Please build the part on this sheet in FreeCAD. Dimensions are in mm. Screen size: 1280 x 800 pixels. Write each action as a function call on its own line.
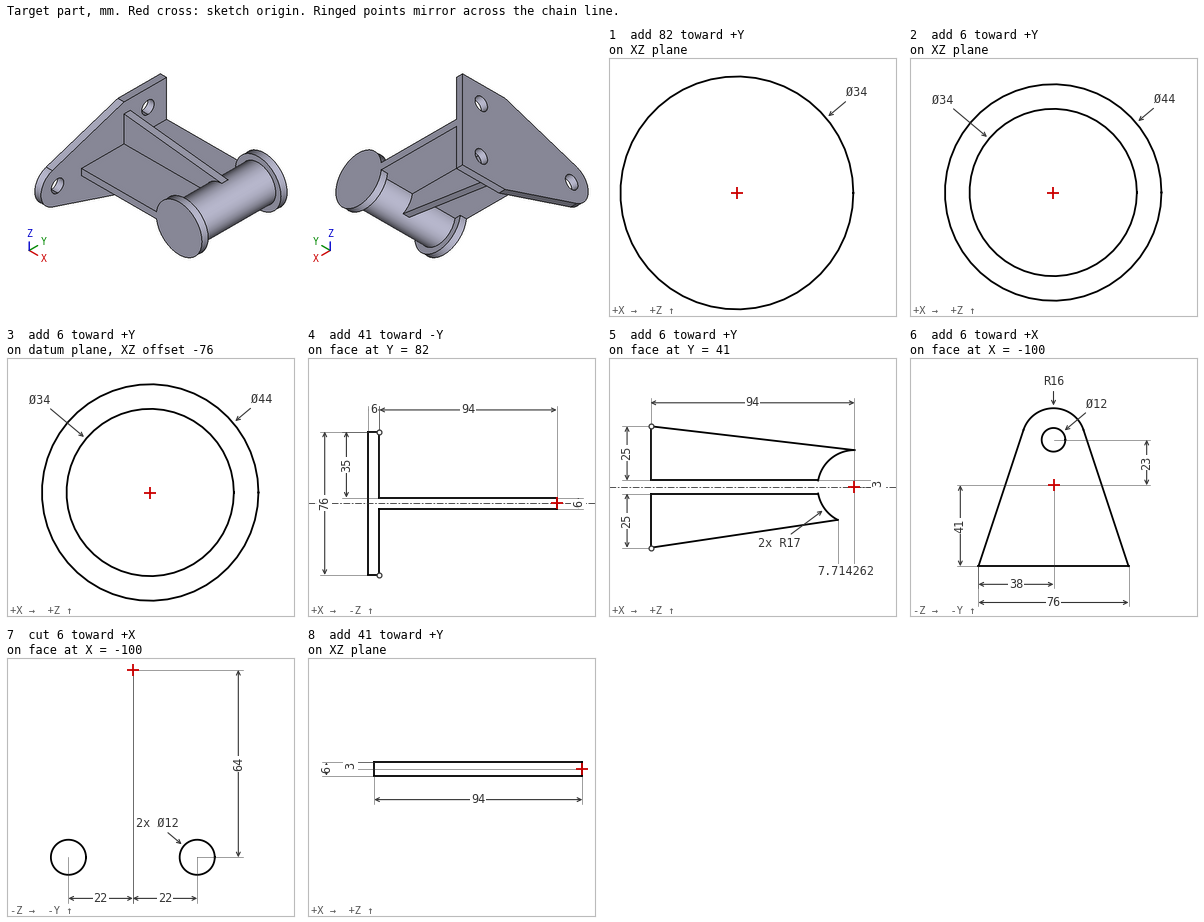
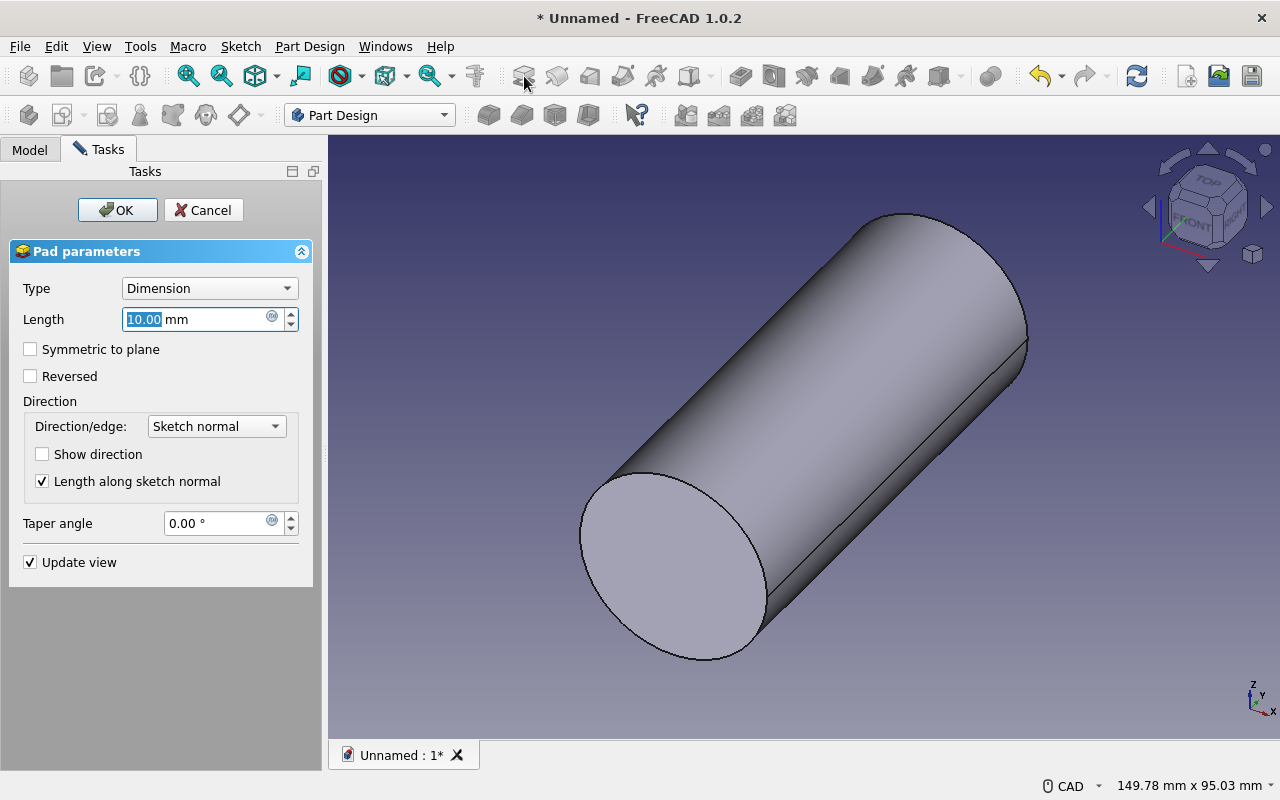
text(6)
key(Tab)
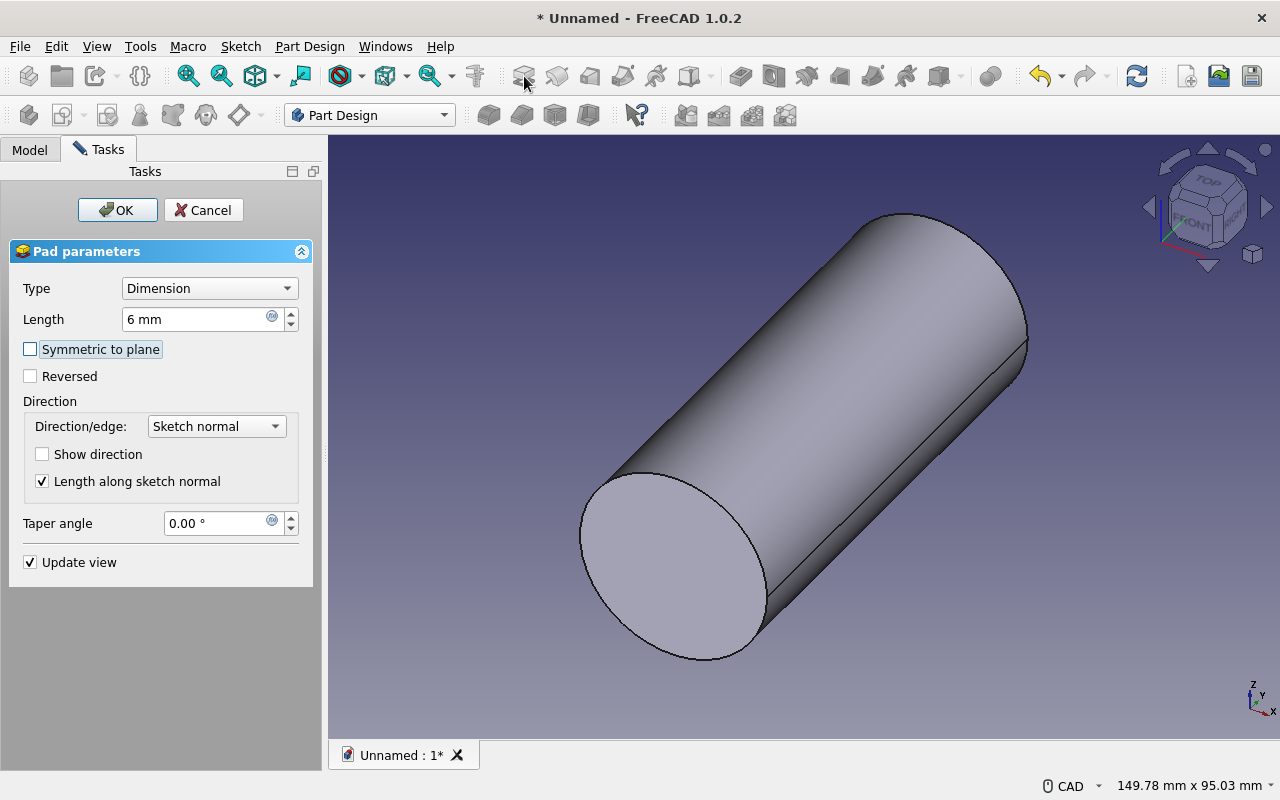
click(31, 376)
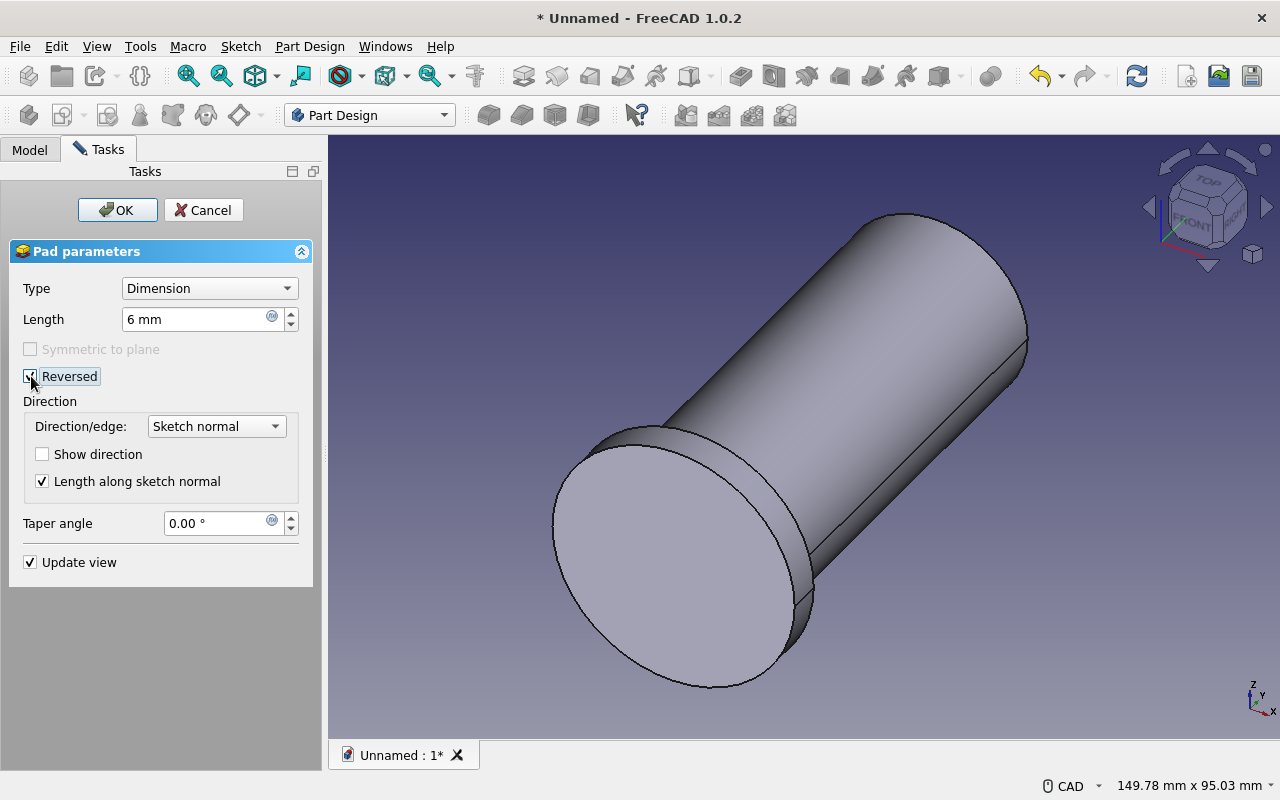
click(118, 210)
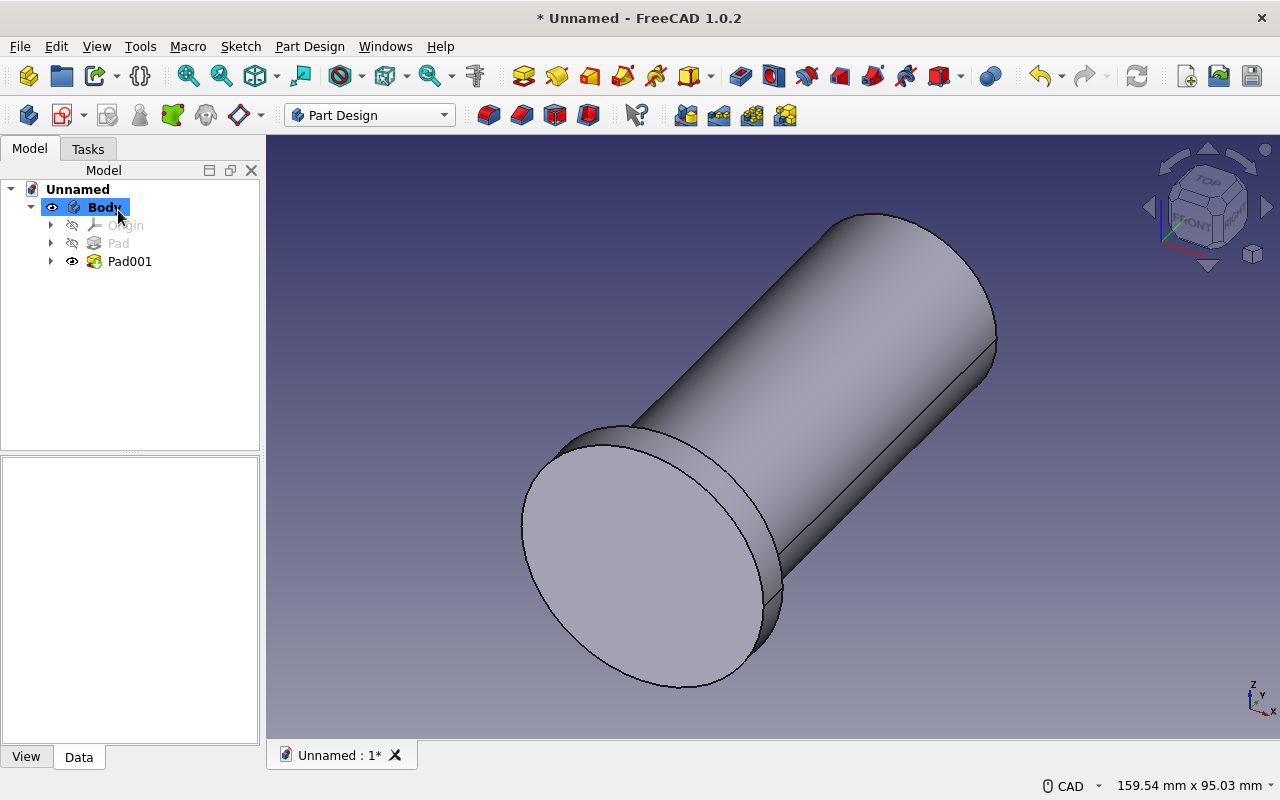
click(51, 225)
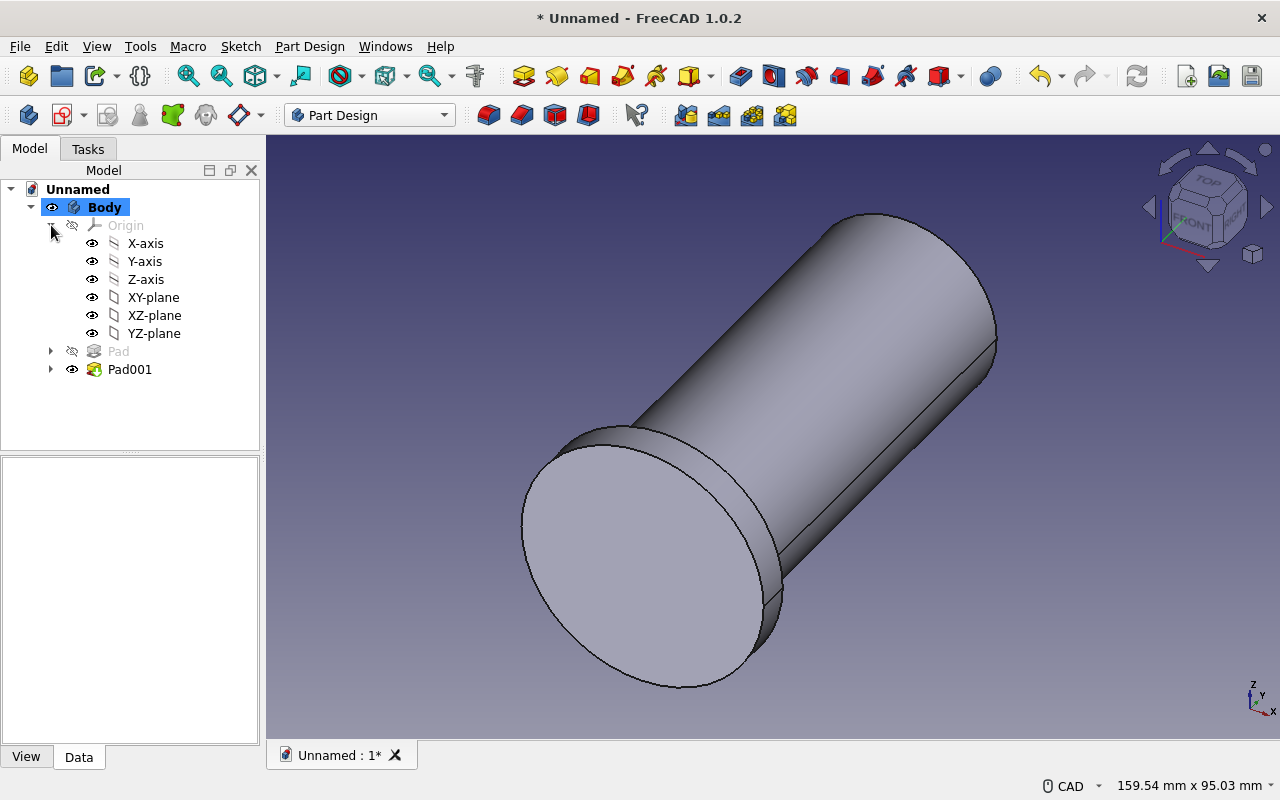
click(137, 315)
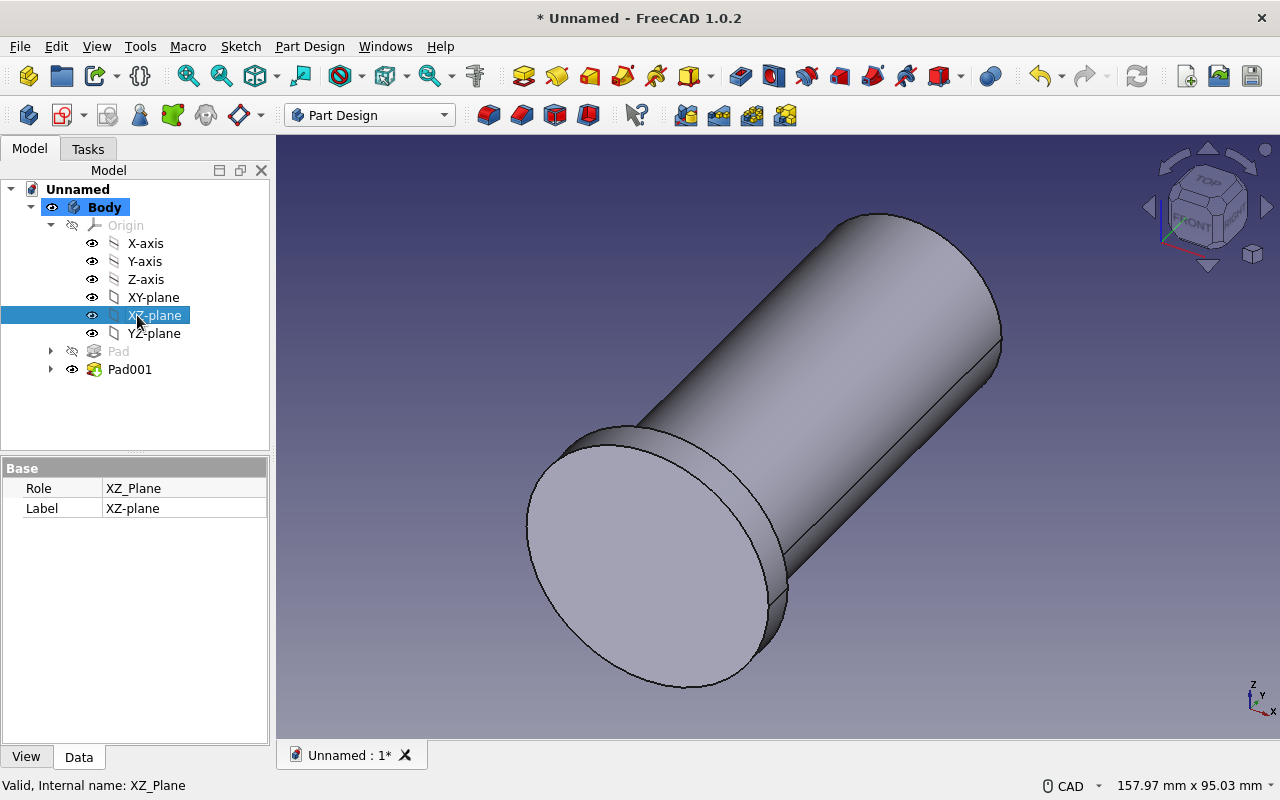
click(238, 116)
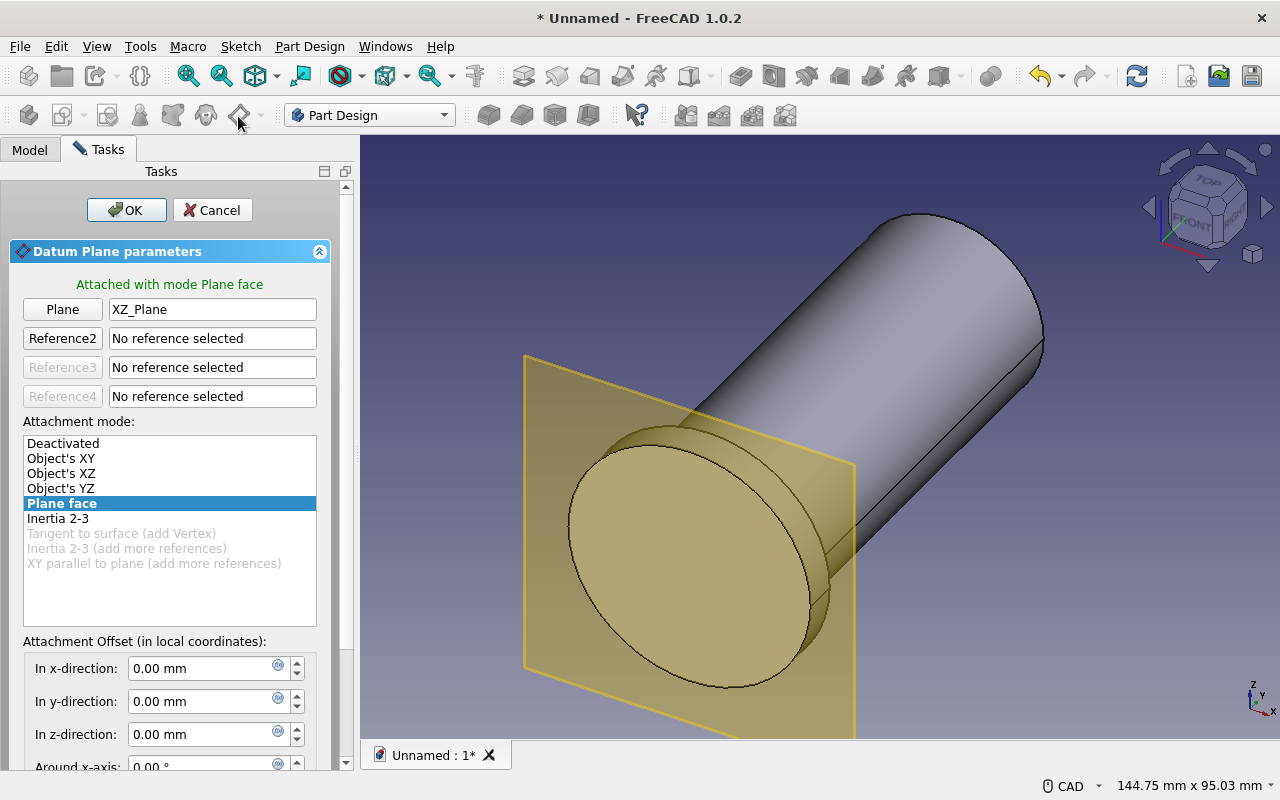
triple_click(210, 734)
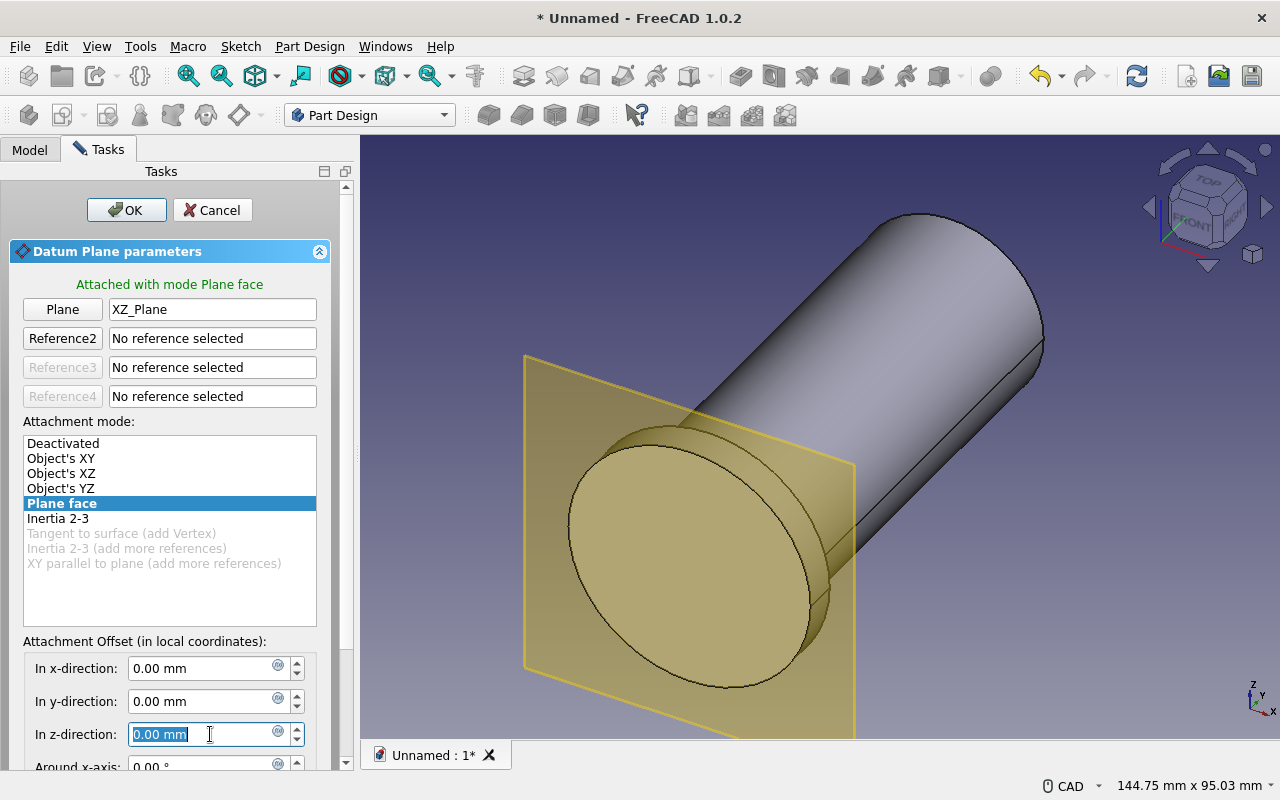
text(-76)
key(Tab)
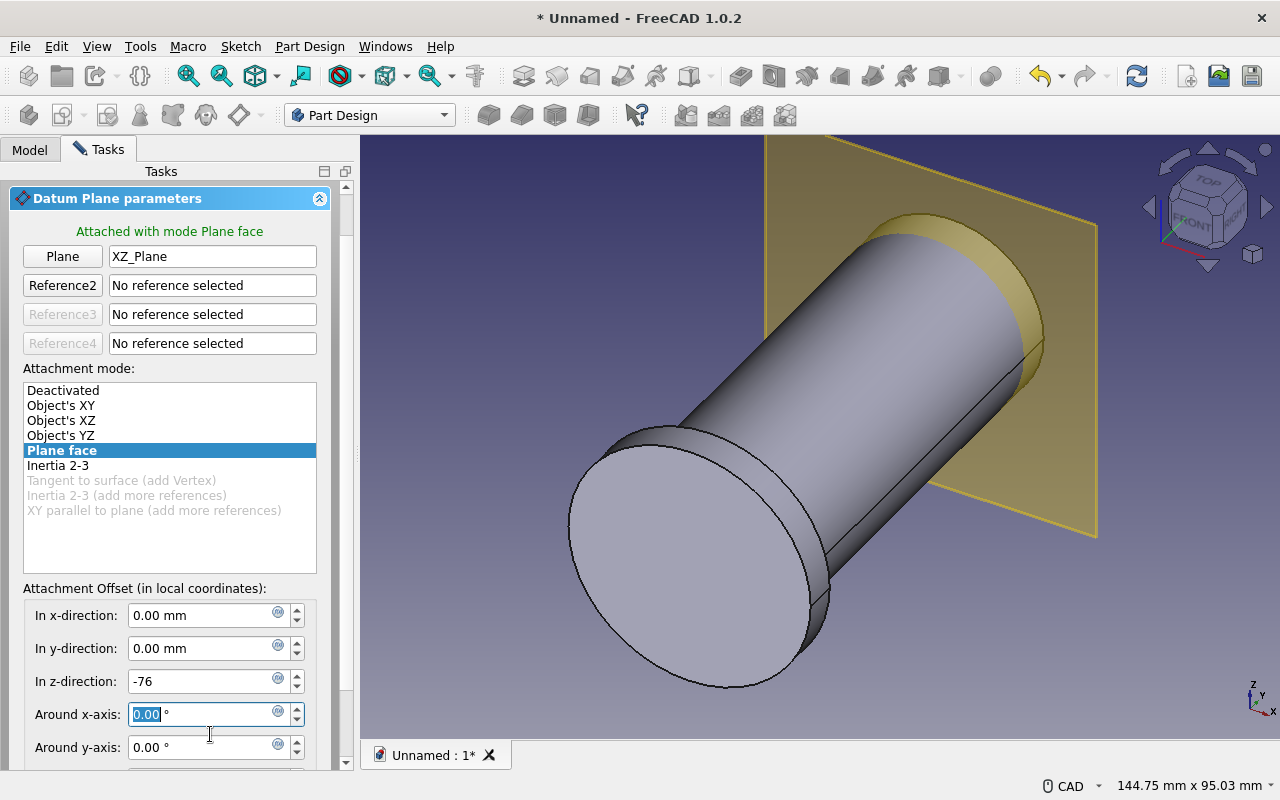
scroll(346, 476, up, 2)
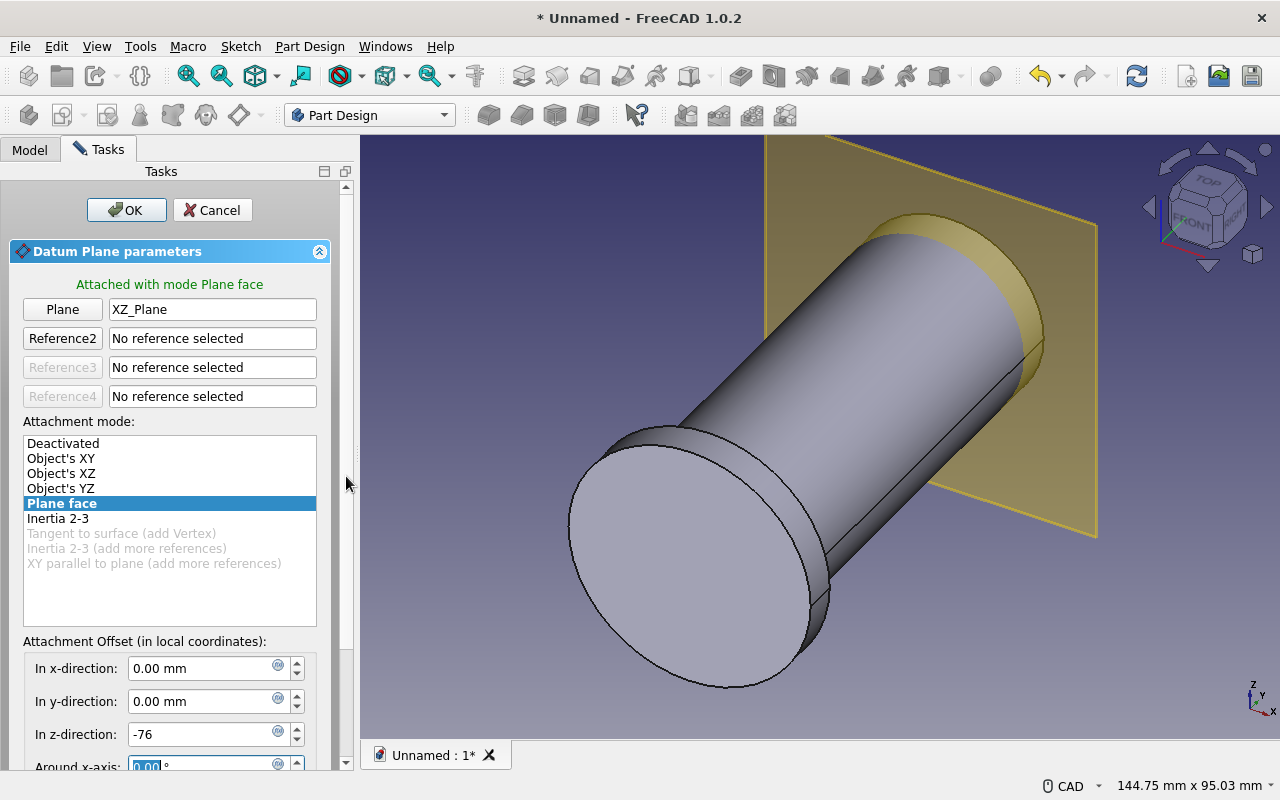
click(127, 210)